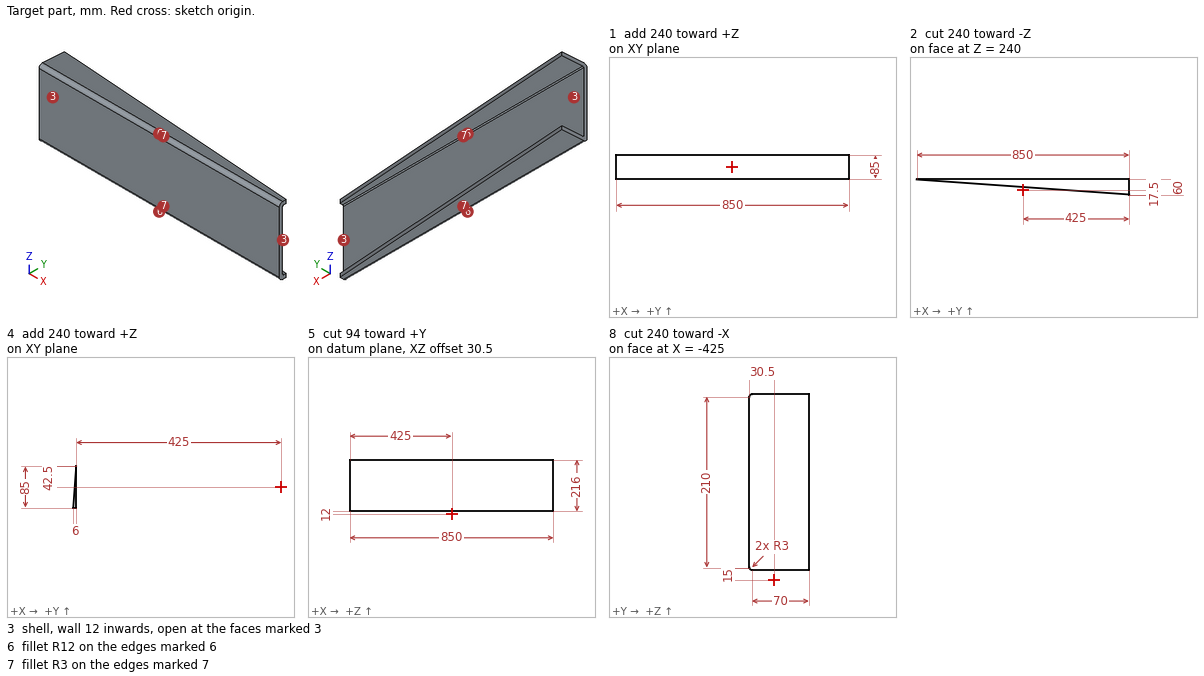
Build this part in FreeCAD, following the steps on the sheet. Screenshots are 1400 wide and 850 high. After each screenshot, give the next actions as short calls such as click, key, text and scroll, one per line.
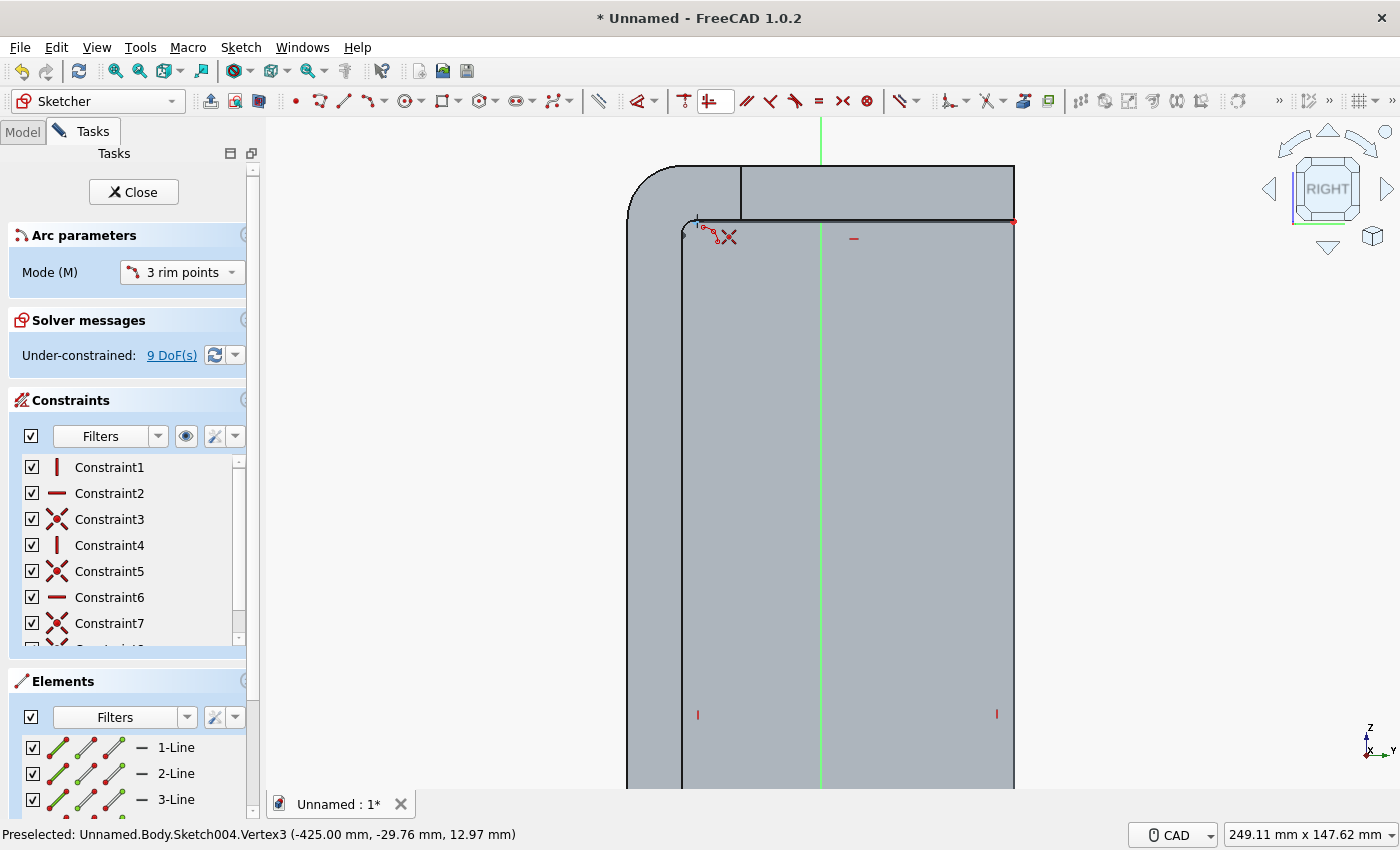
click(696, 222)
click(682, 236)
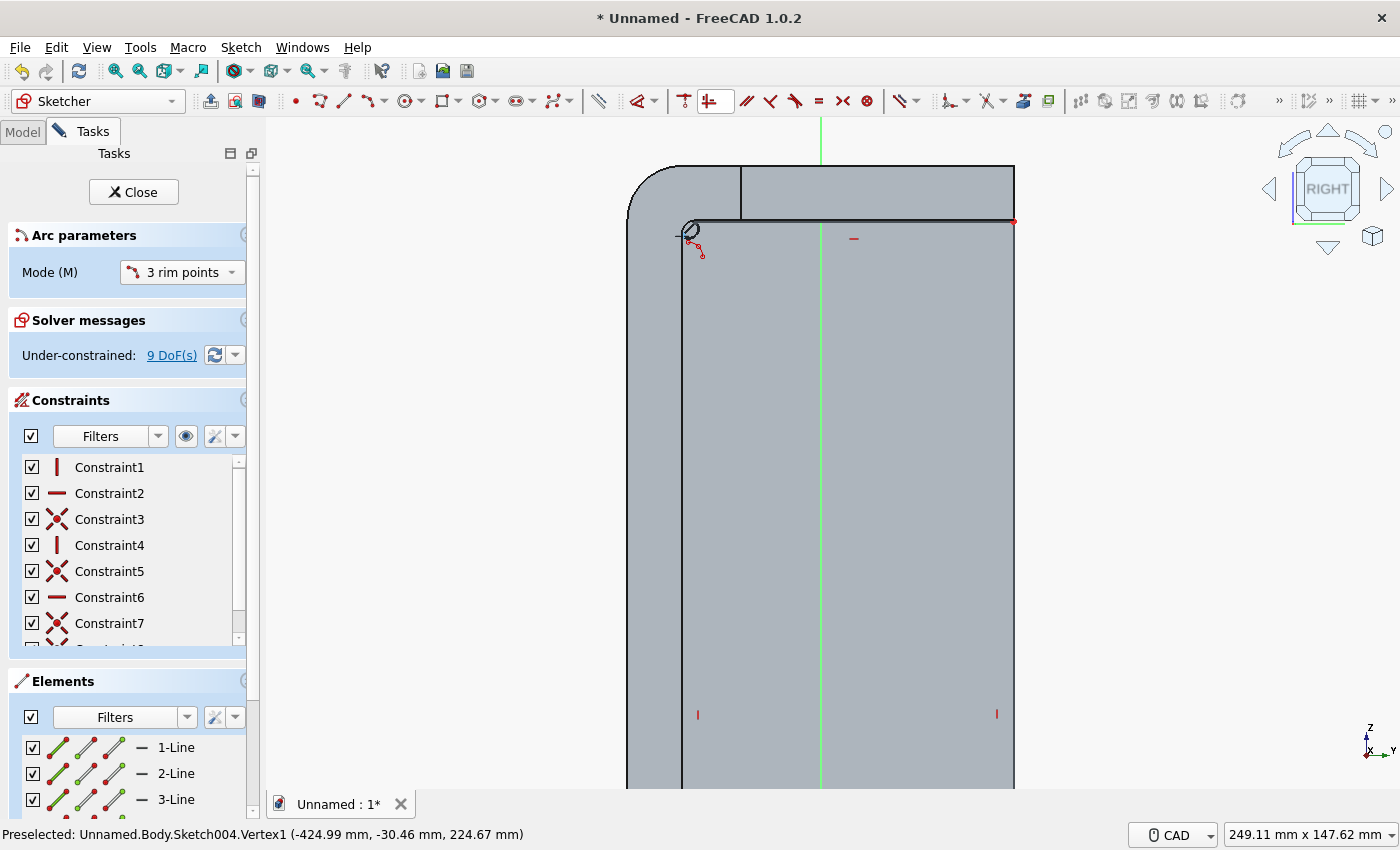
scroll(686, 224, up, 7)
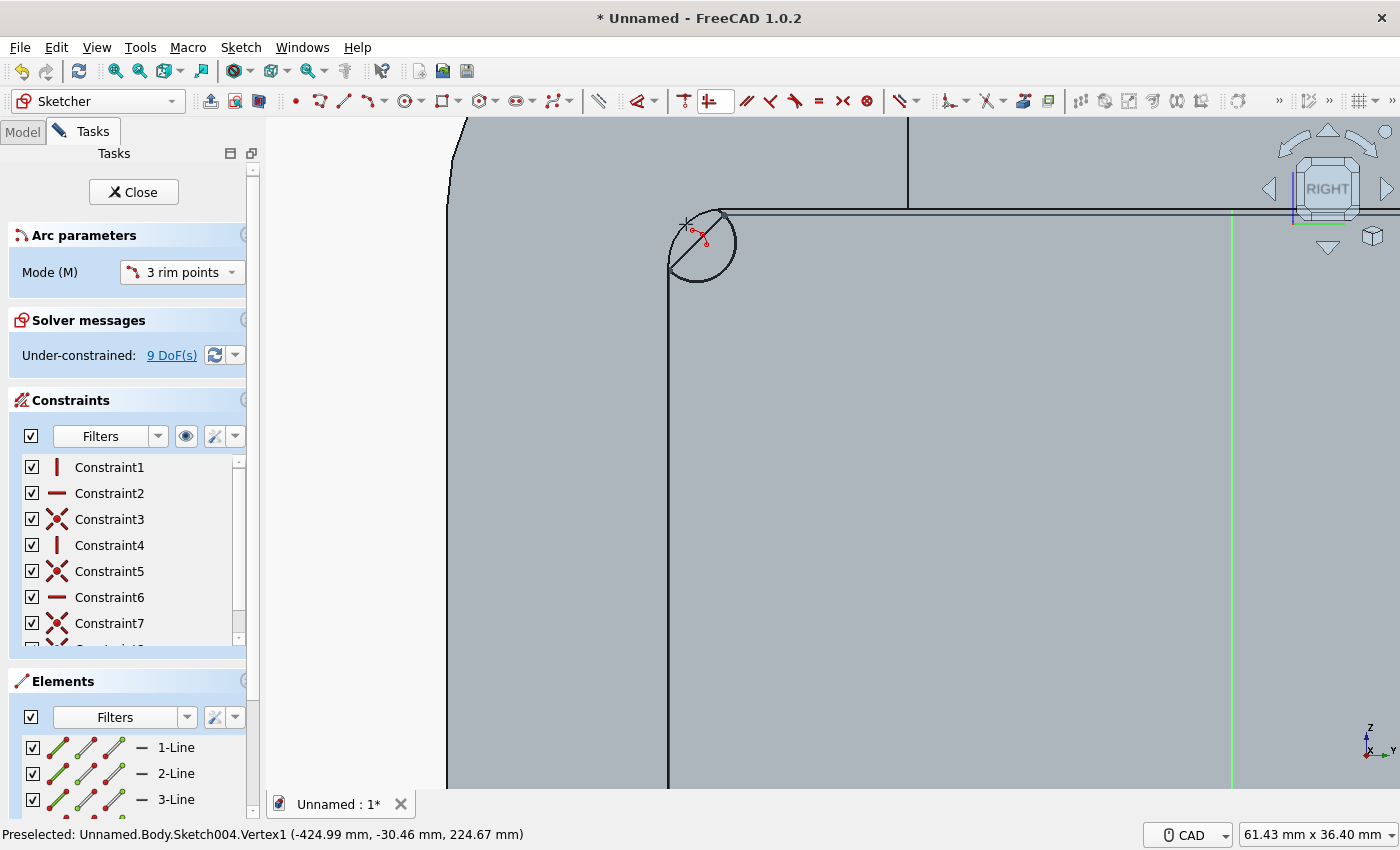
click(685, 225)
key(Escape)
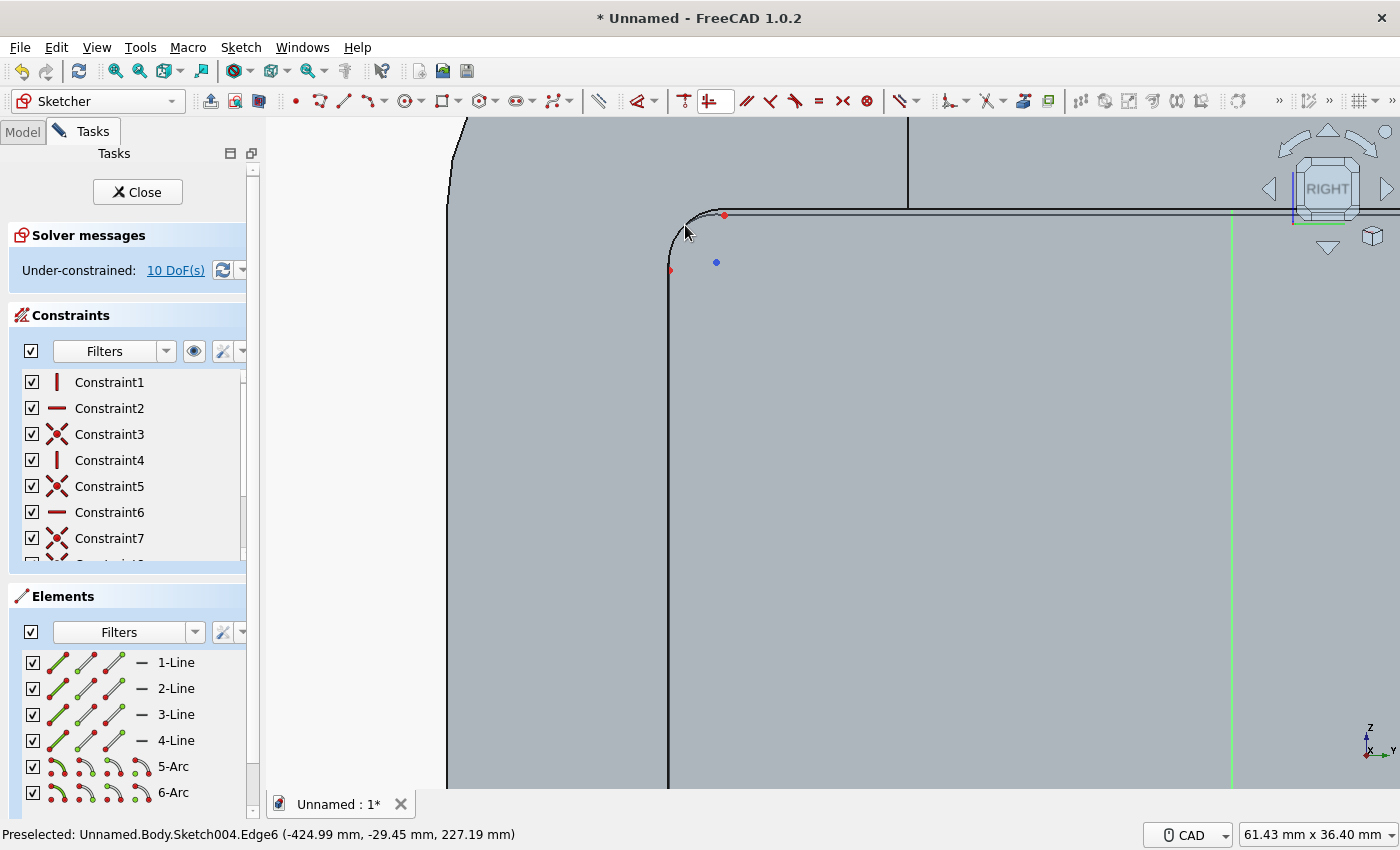
scroll(693, 221, down, 11)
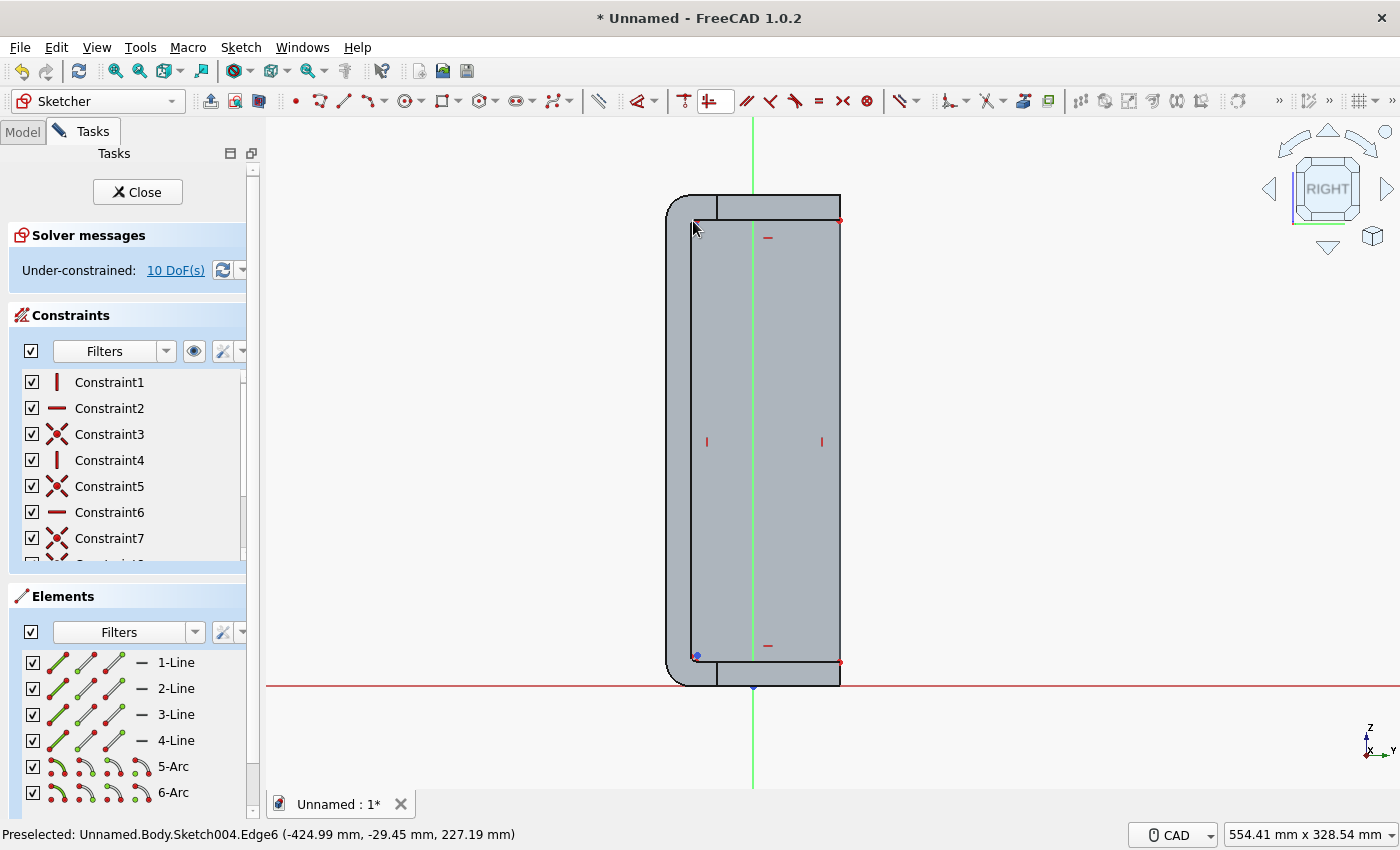
click(691, 356)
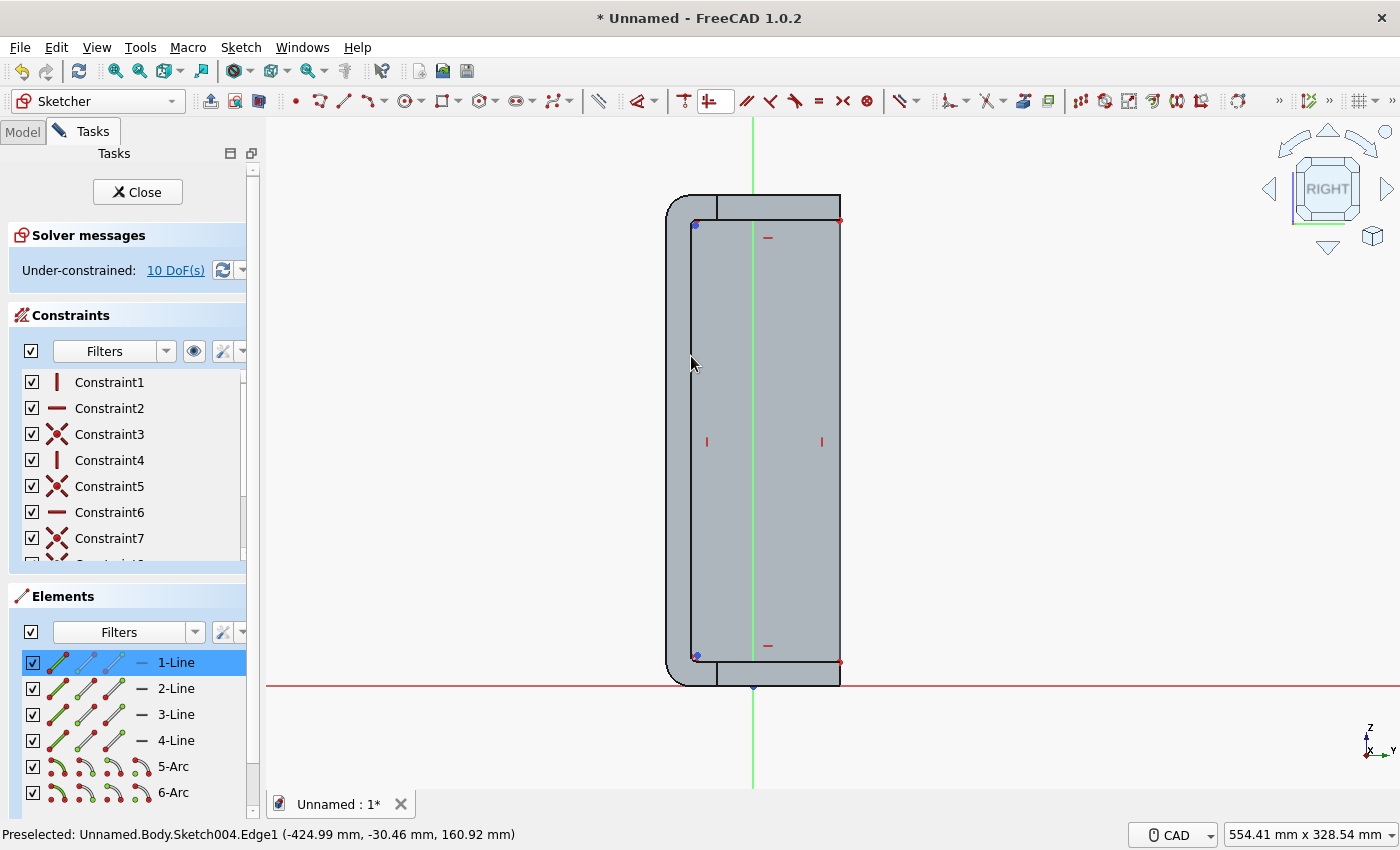
scroll(693, 660, up, 6)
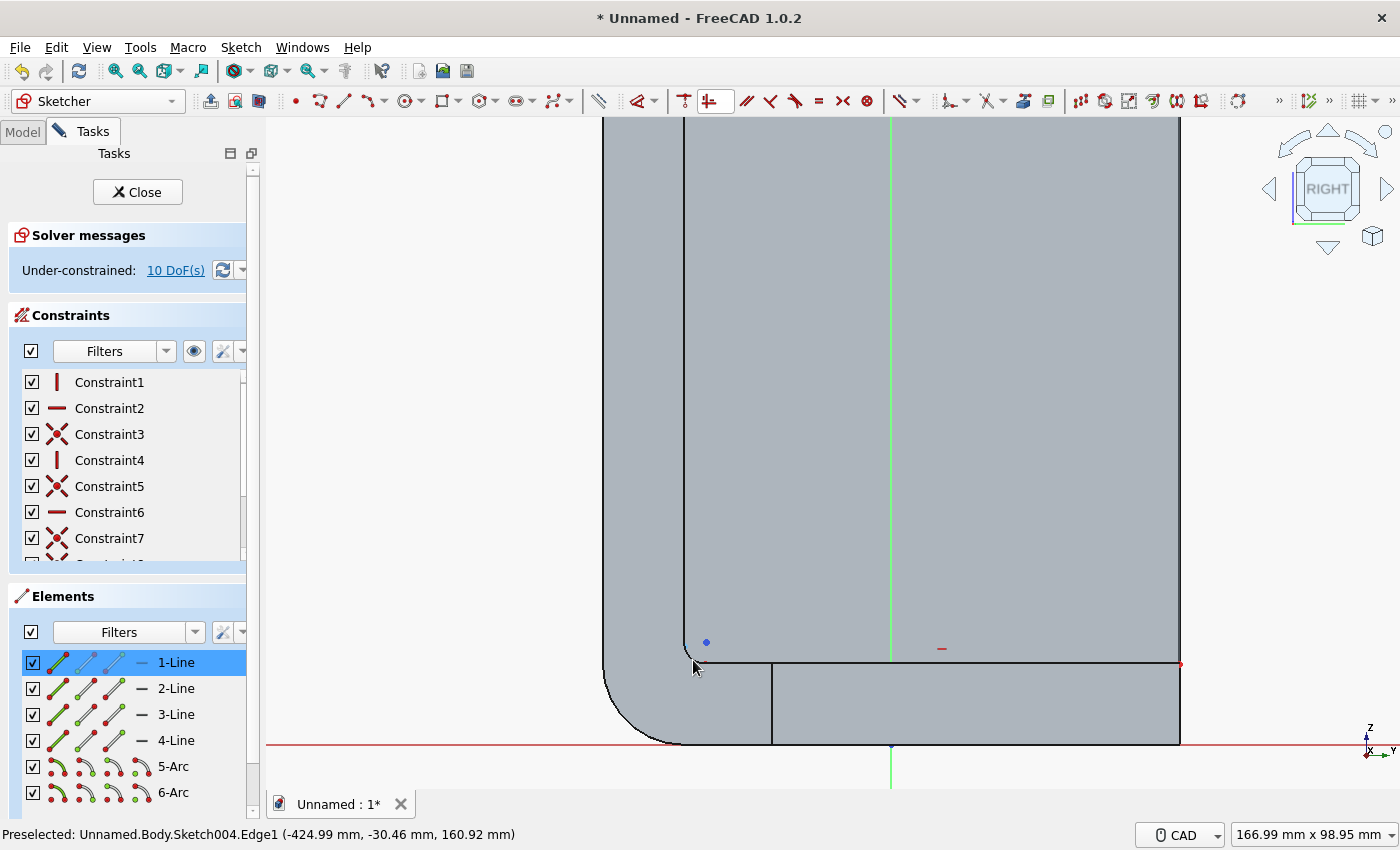
click(692, 659)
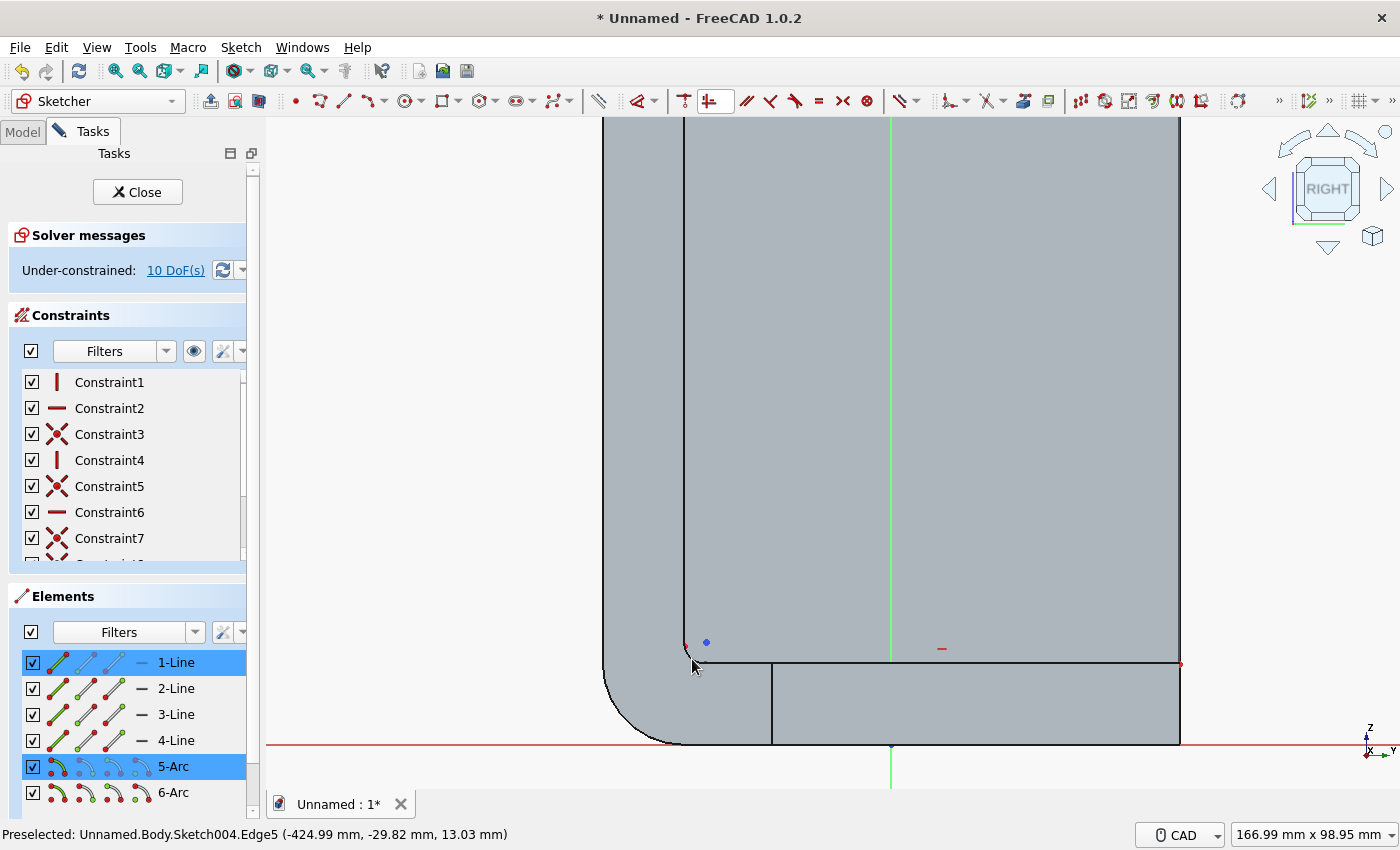
key(t)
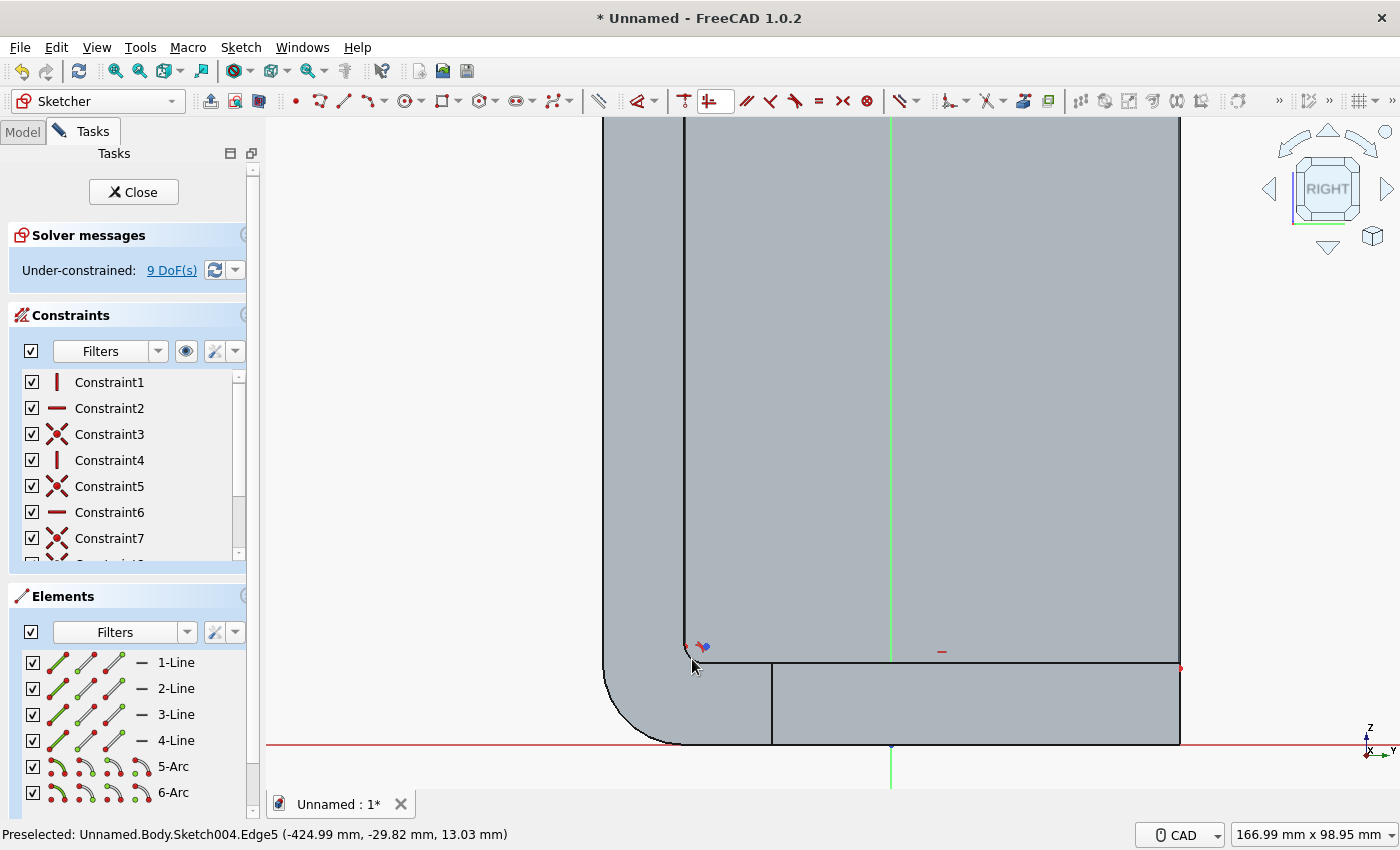
click(685, 218)